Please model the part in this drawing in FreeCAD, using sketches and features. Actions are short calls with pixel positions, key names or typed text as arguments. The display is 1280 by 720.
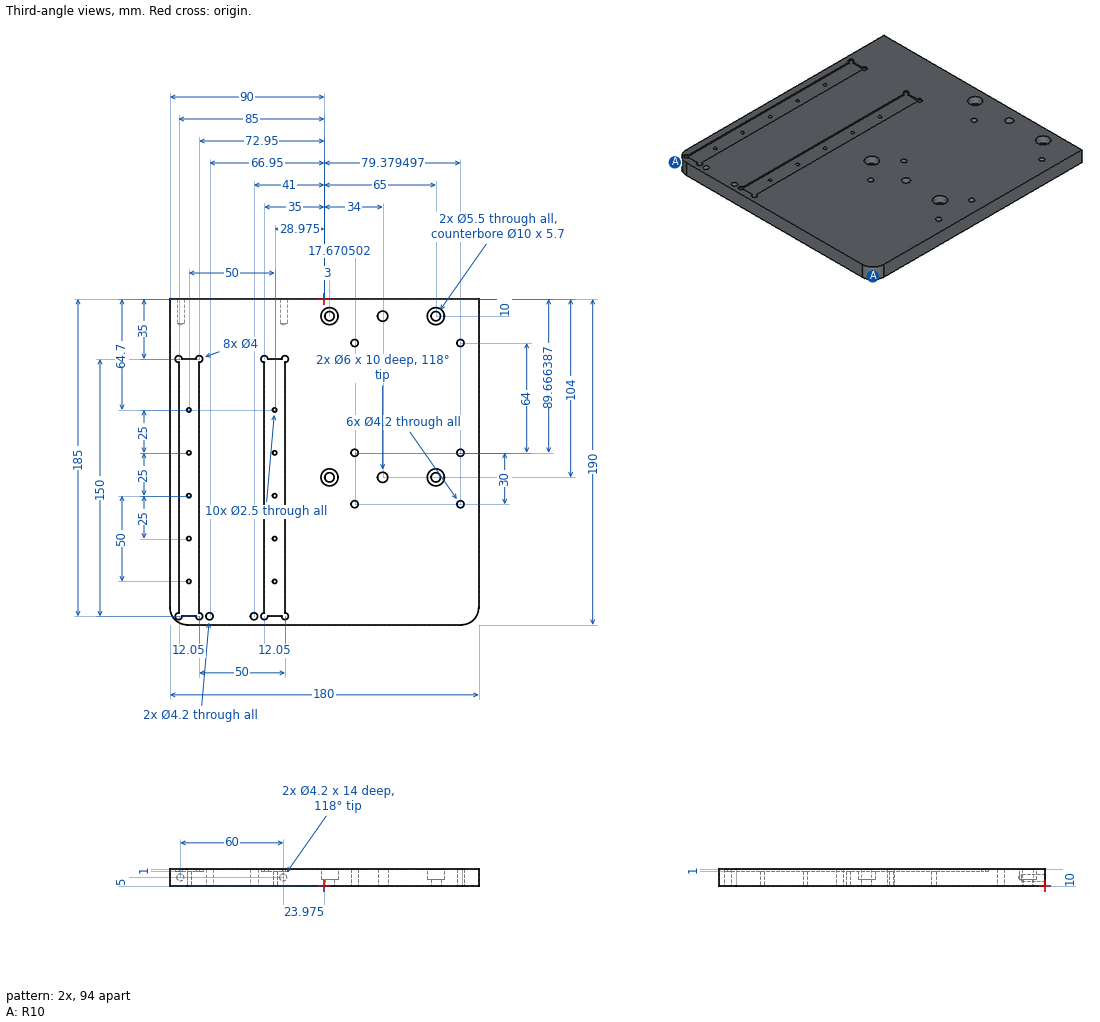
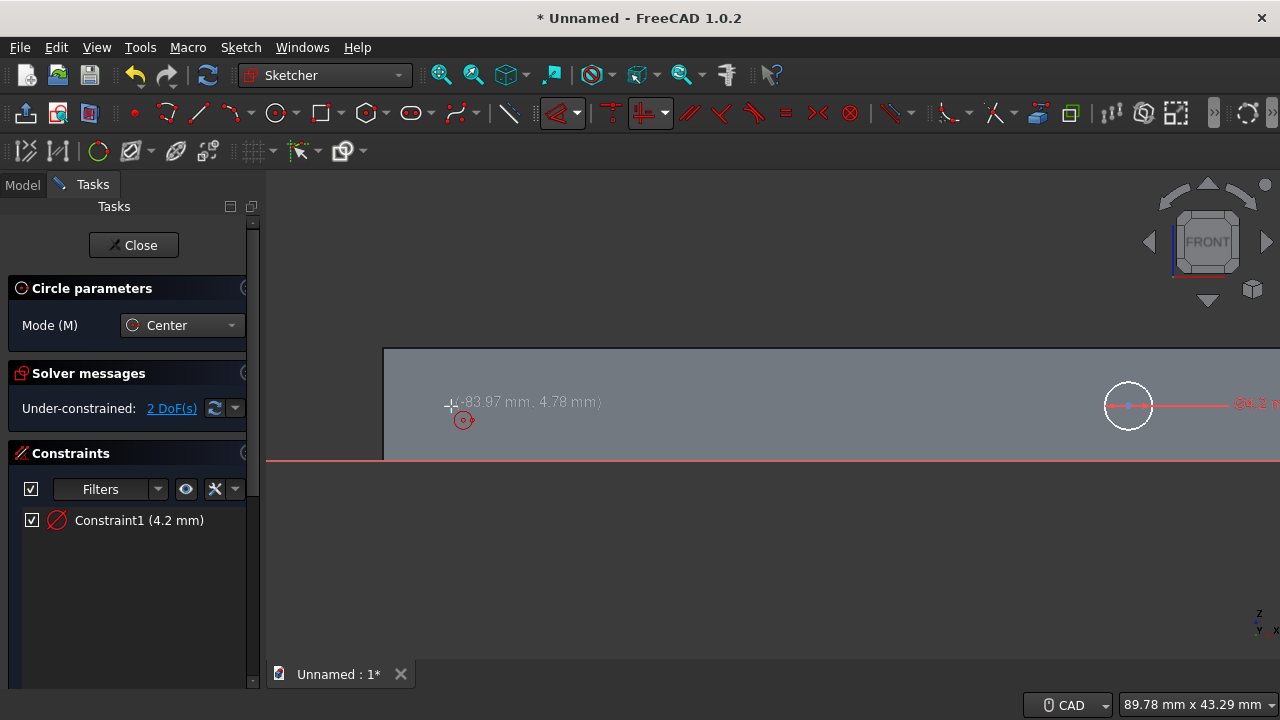
click(451, 405)
move(468, 388)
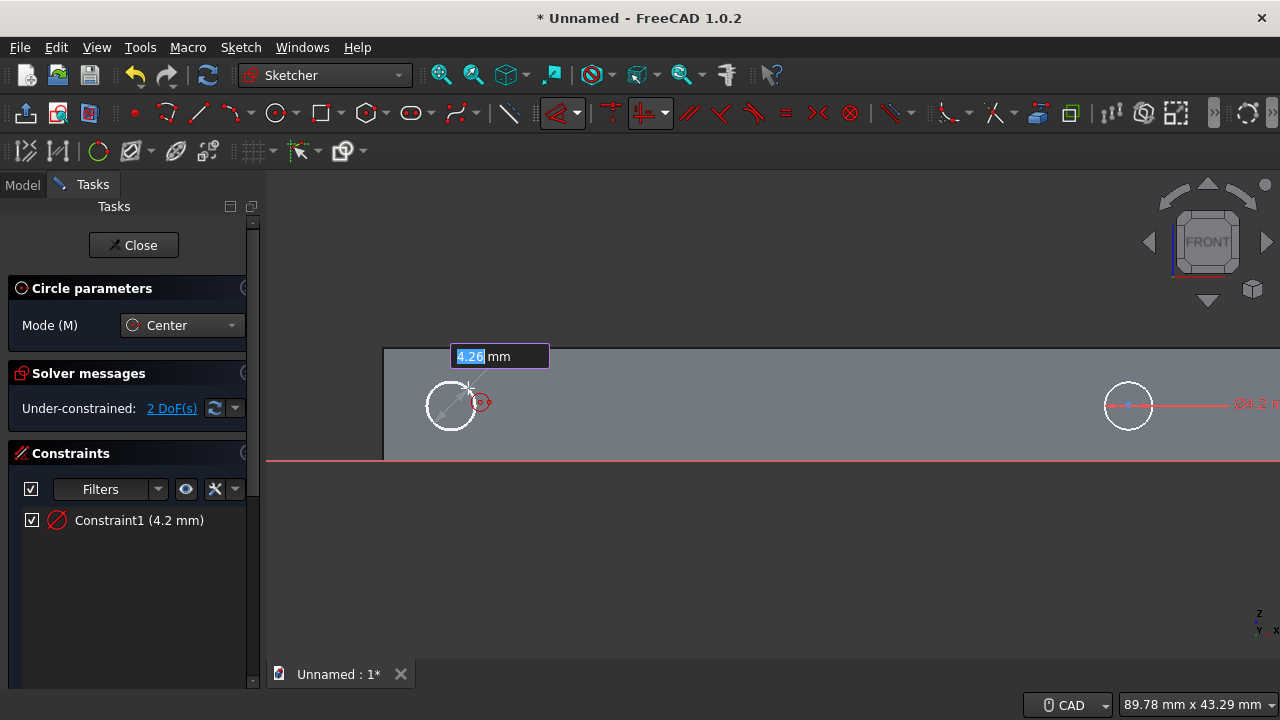
text(4.2)
key(Return)
key(Escape)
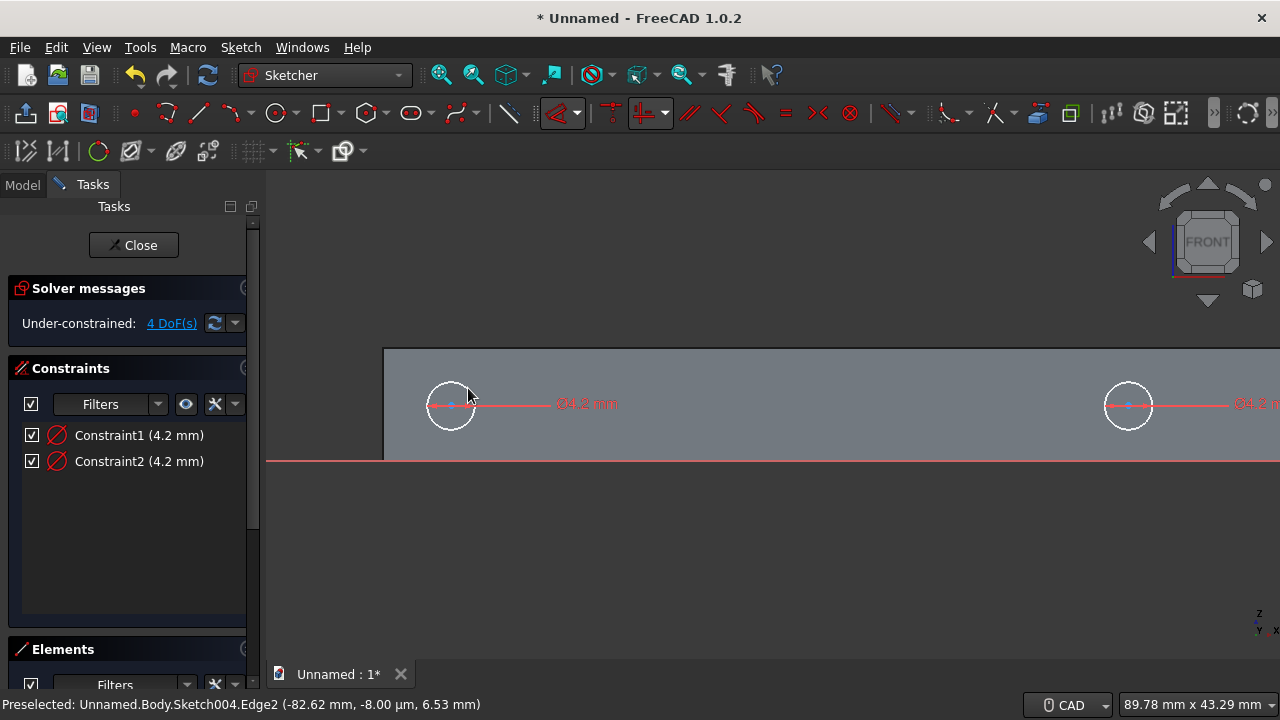
scroll(451, 406, down, 3)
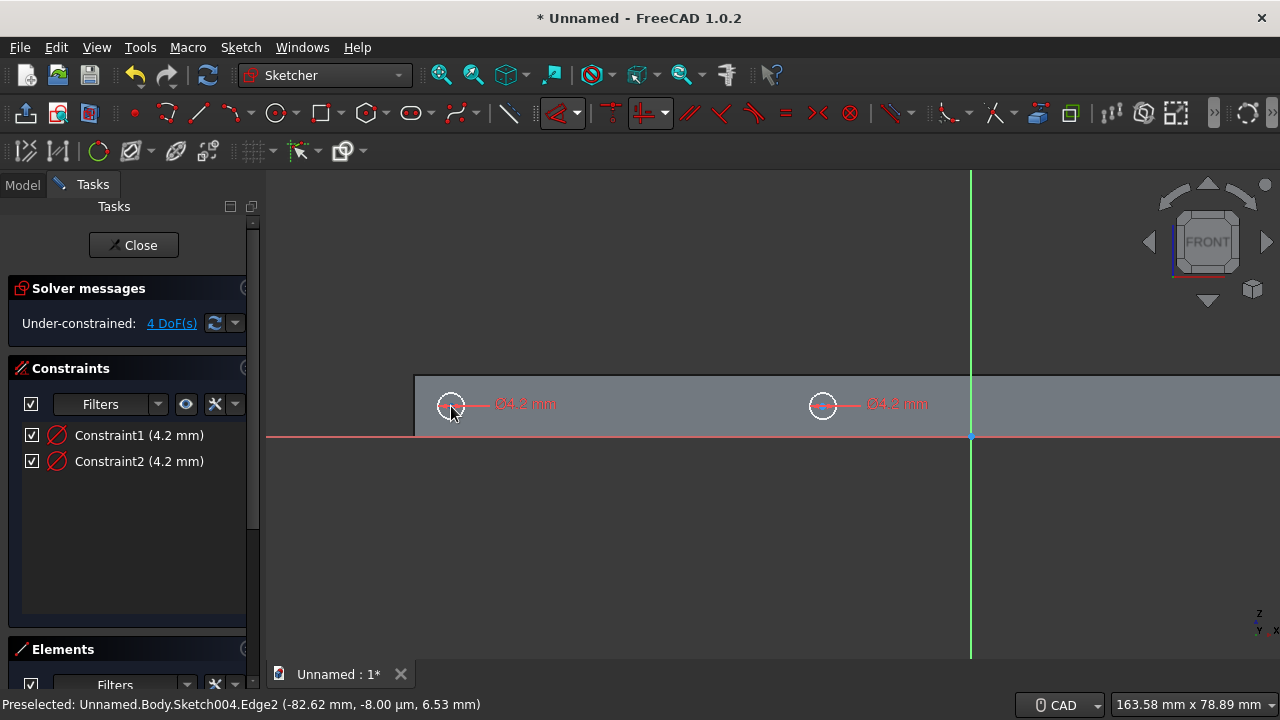
click(823, 406)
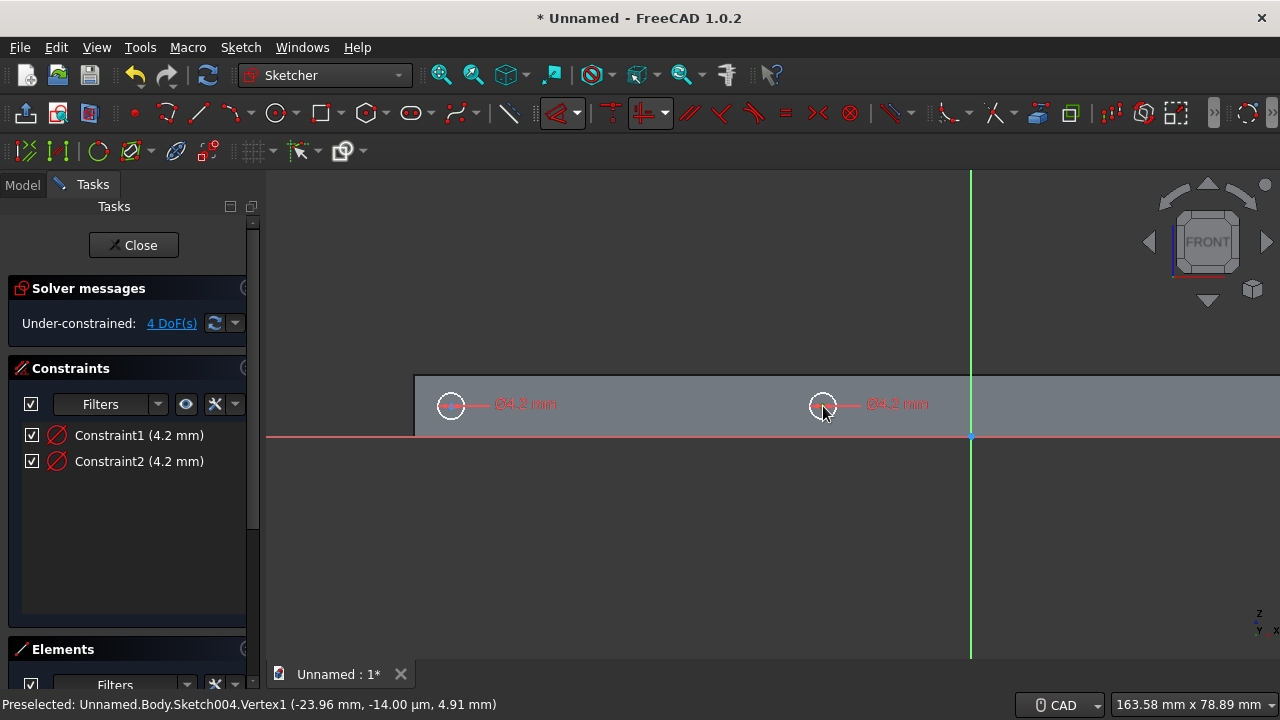
click(451, 406)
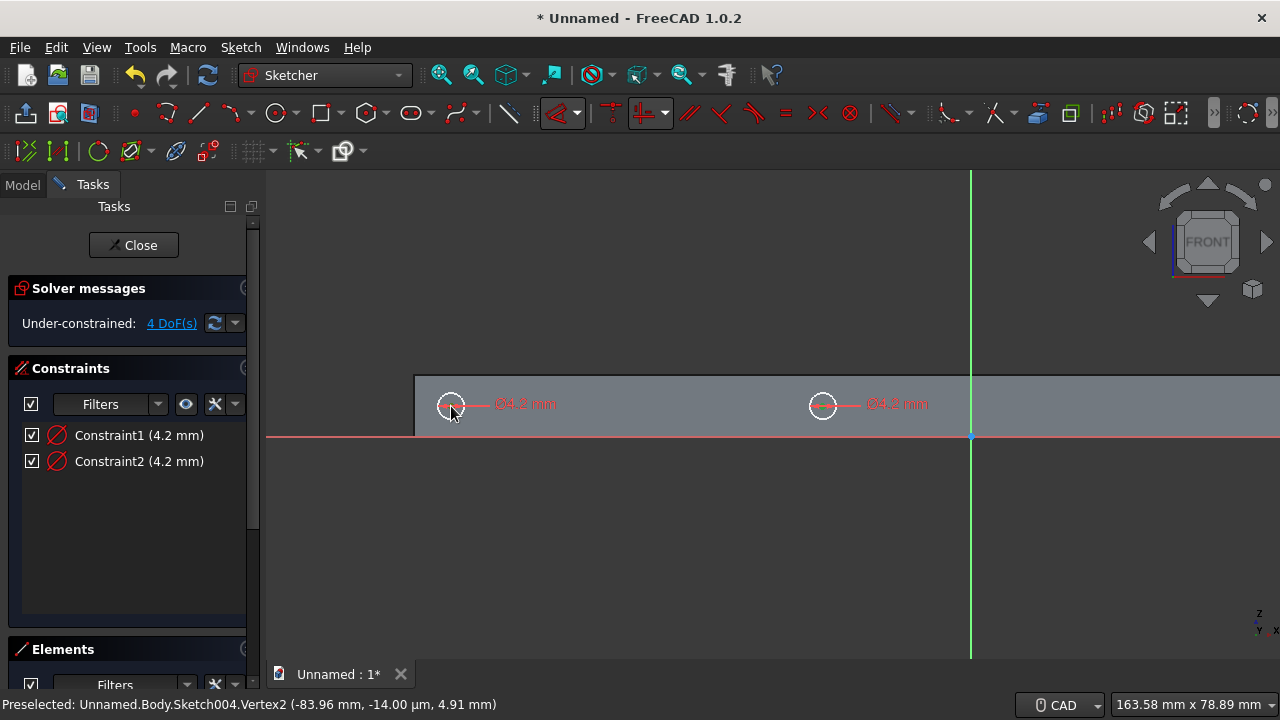
key(h)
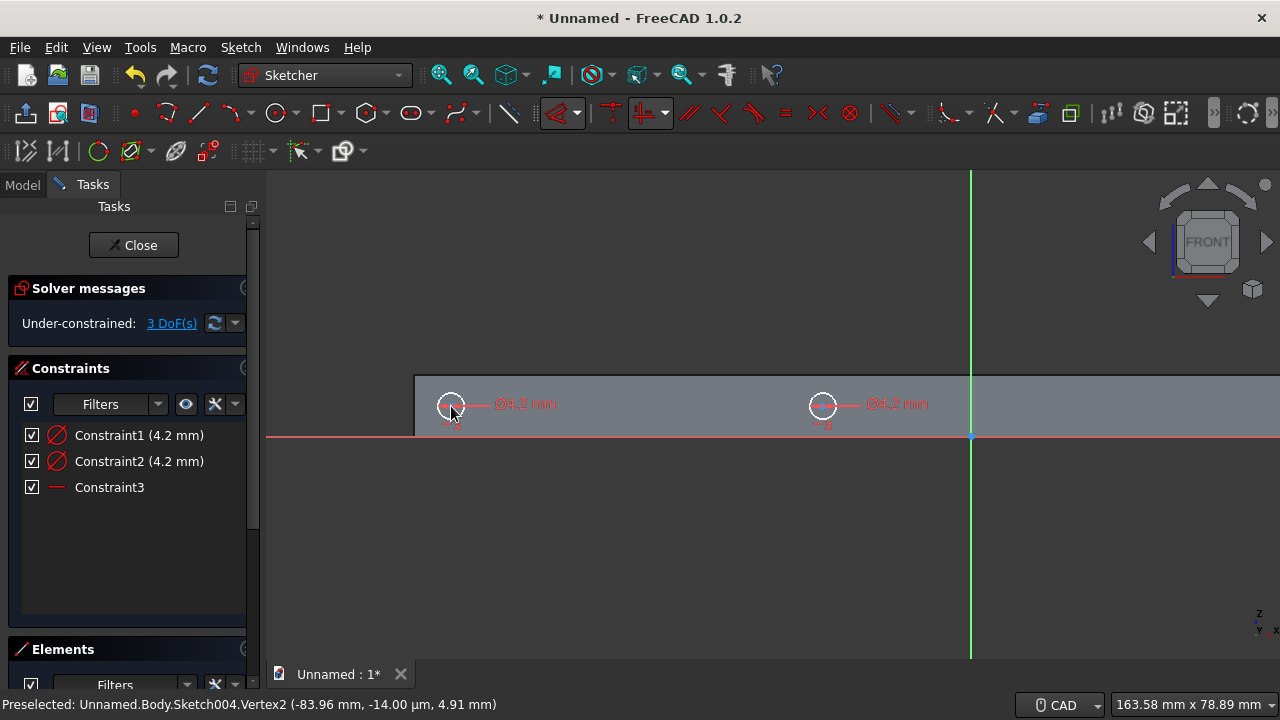
scroll(823, 406, up, 2)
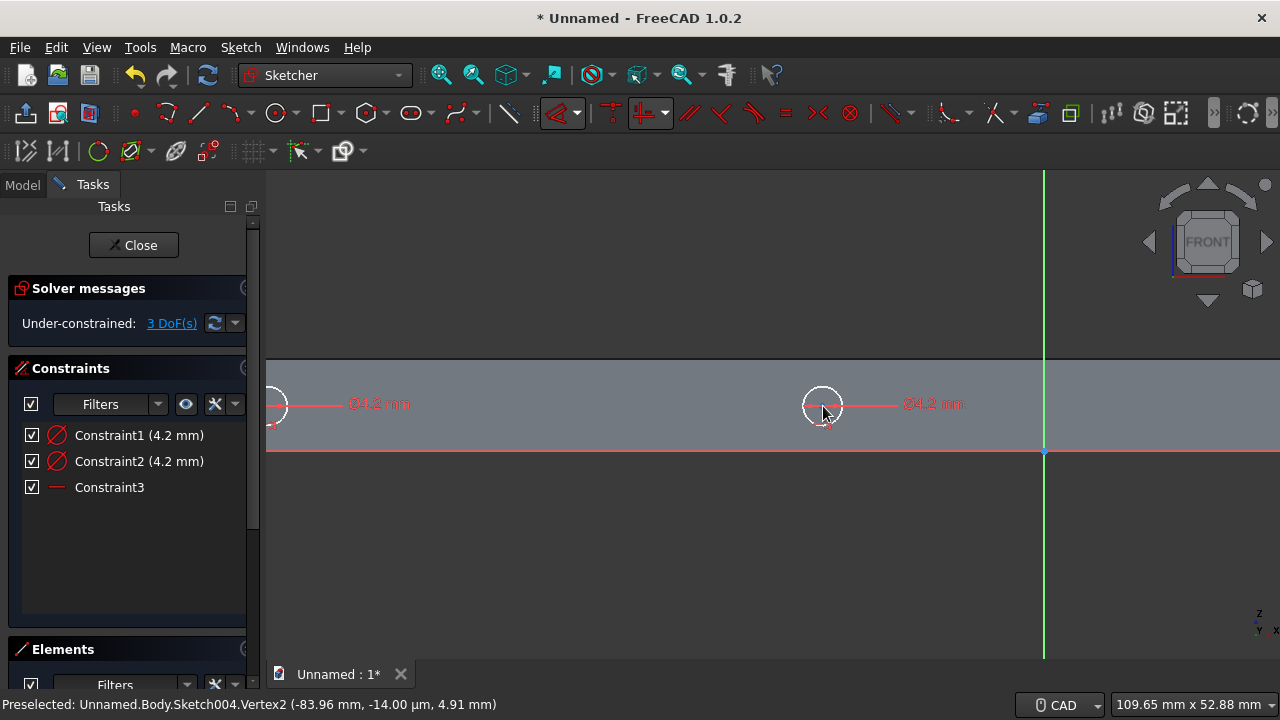
click(823, 406)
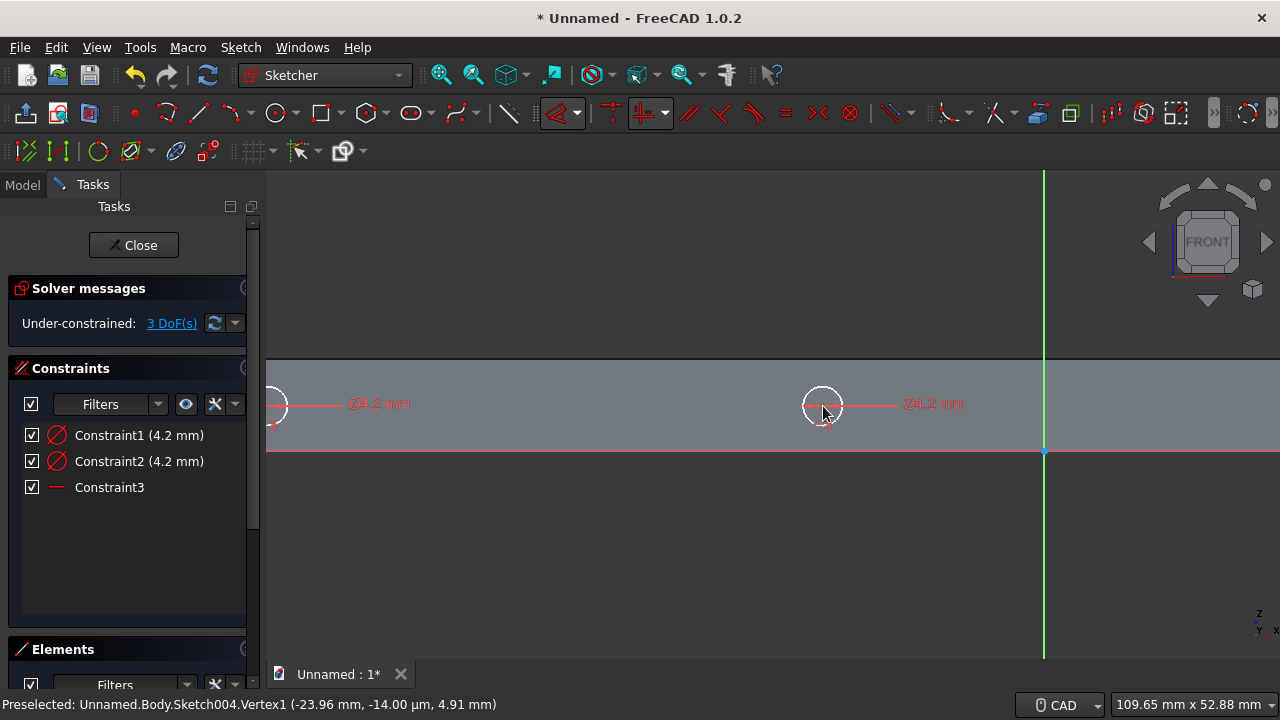
key(i)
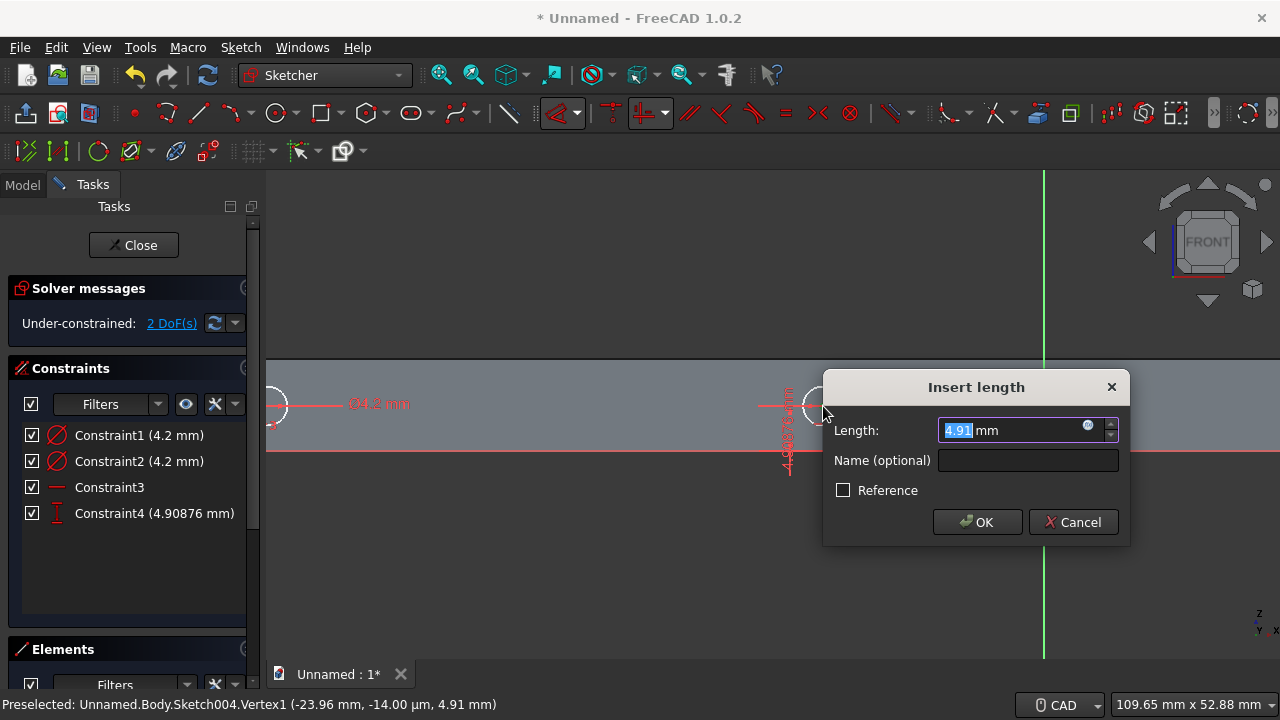
text(5)
key(Return)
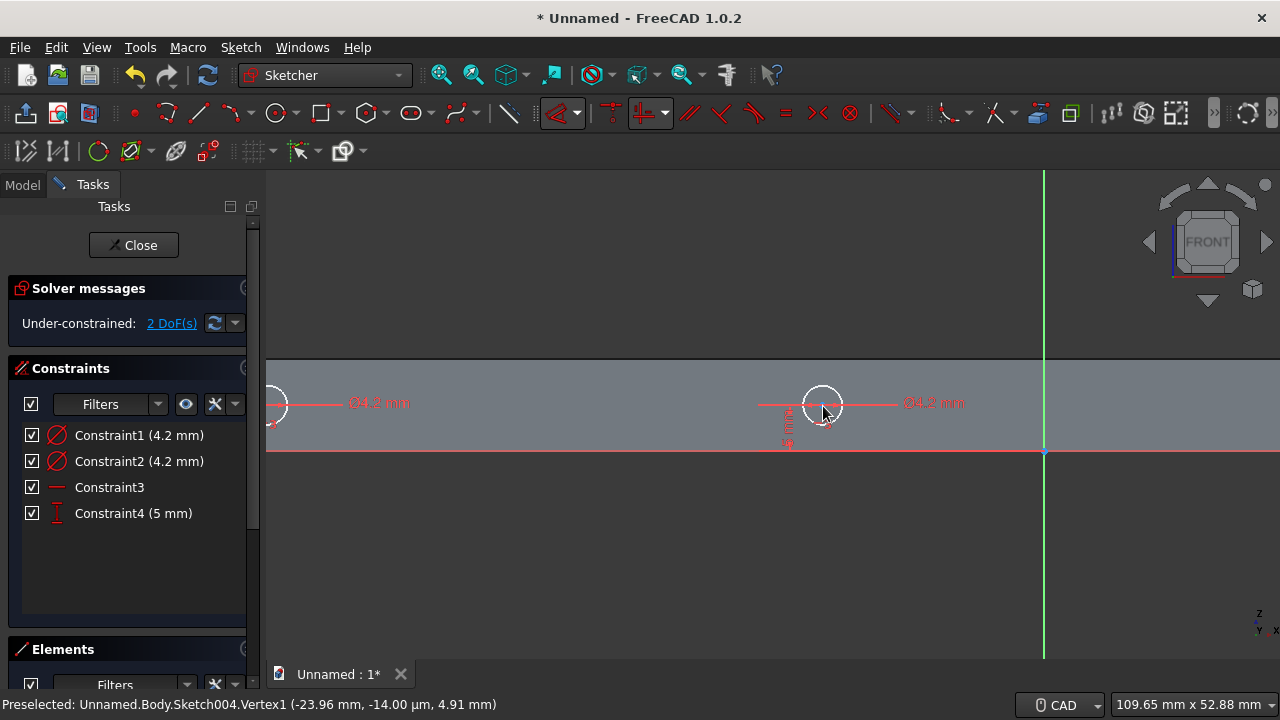
click(823, 405)